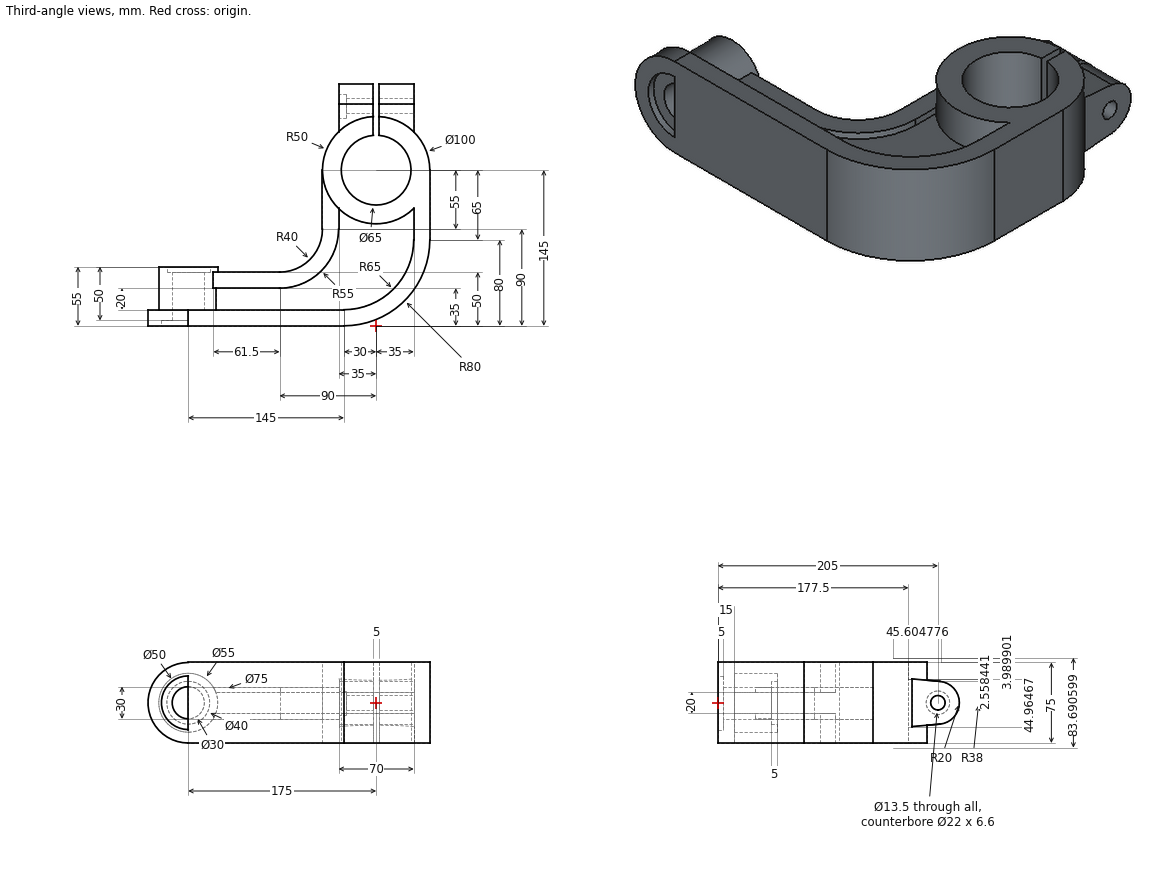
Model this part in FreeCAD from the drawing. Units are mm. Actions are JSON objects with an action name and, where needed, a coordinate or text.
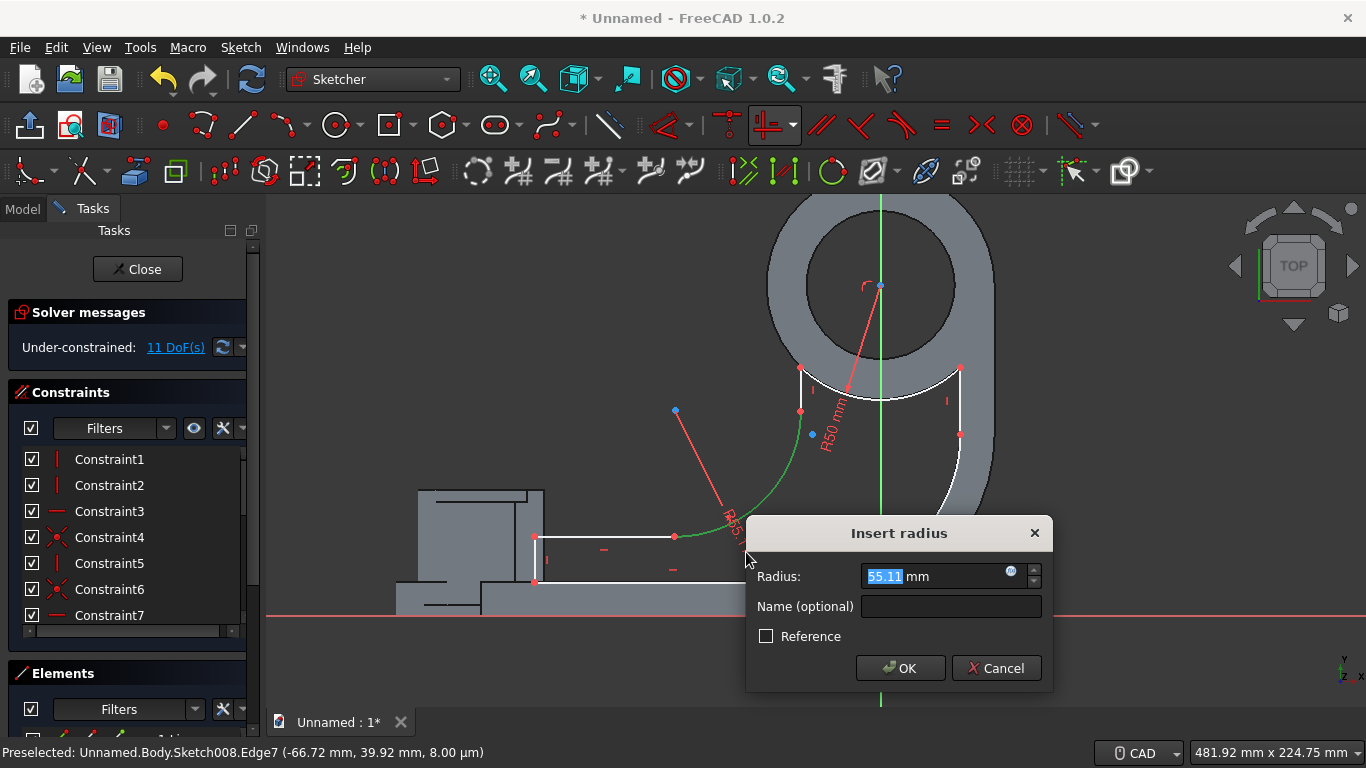
{"action": "type", "text": "55"}
{"action": "key", "text": "Return"}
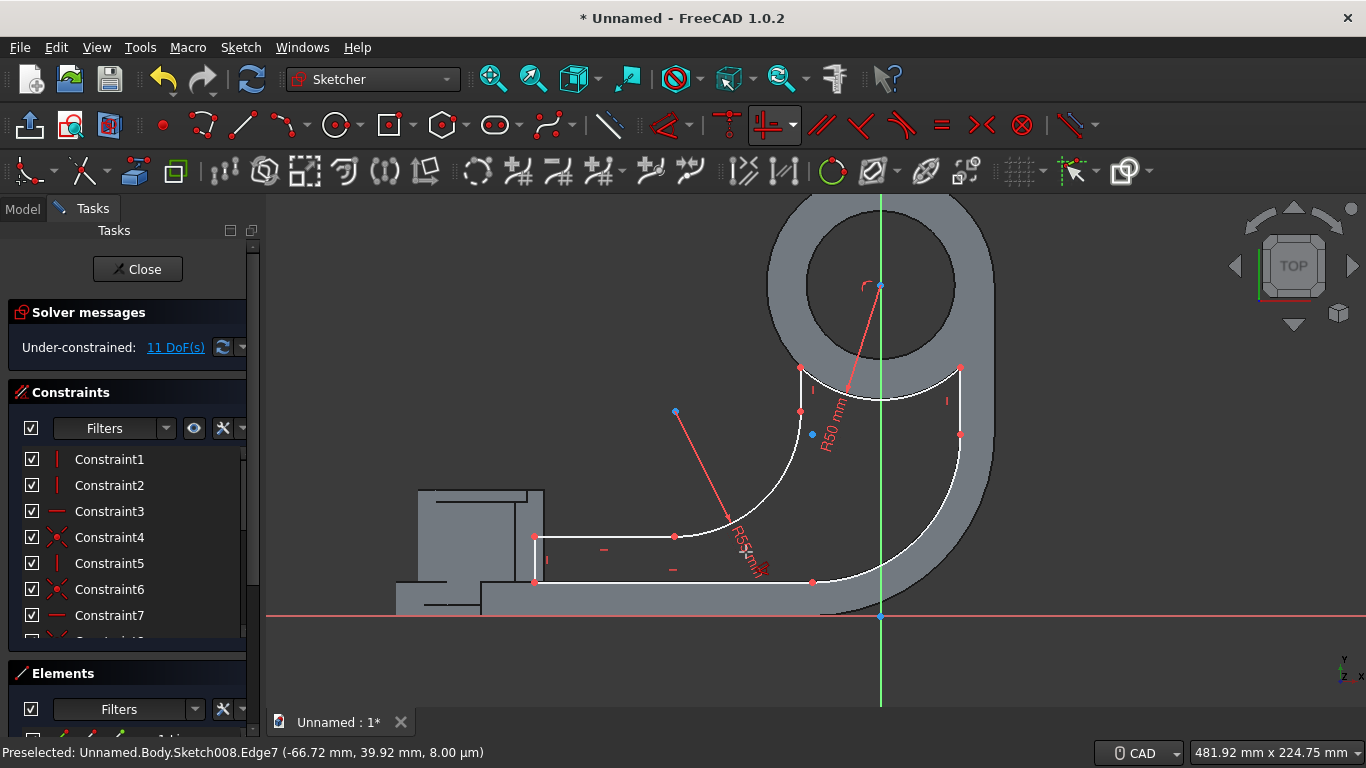
{"action": "left_click", "coordinate": [880, 566]}
{"action": "left_click", "coordinate": [895, 594]}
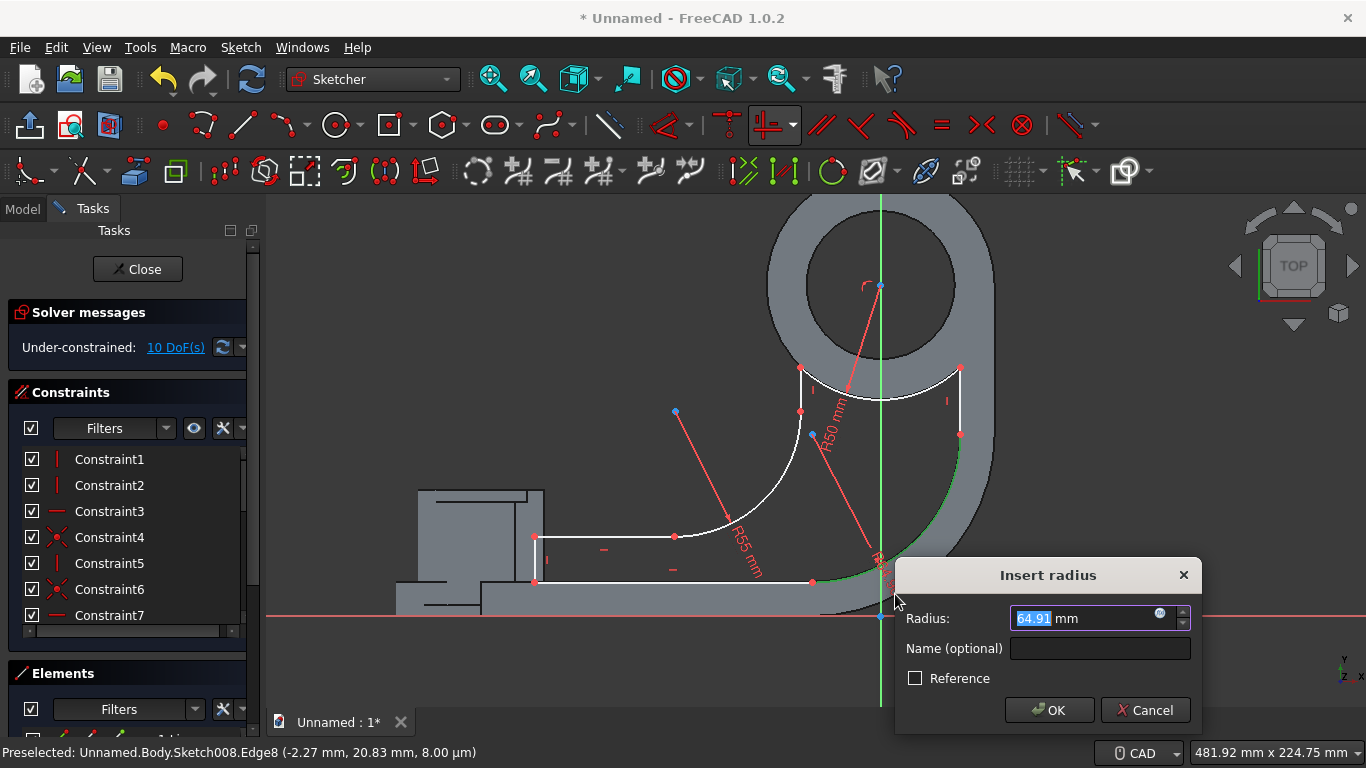
{"action": "type", "text": "65"}
{"action": "key", "text": "Return"}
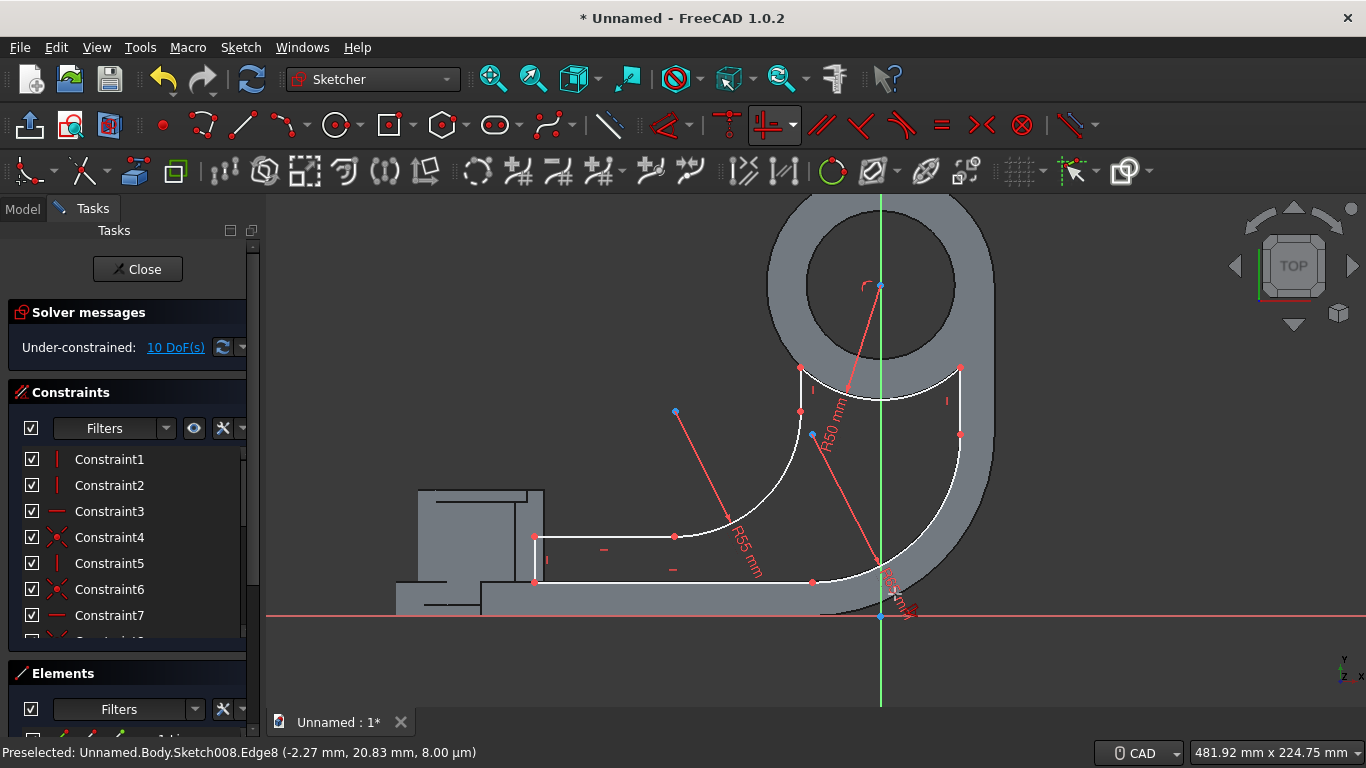
{"action": "left_click", "coordinate": [535, 551]}
{"action": "left_click", "coordinate": [501, 560]}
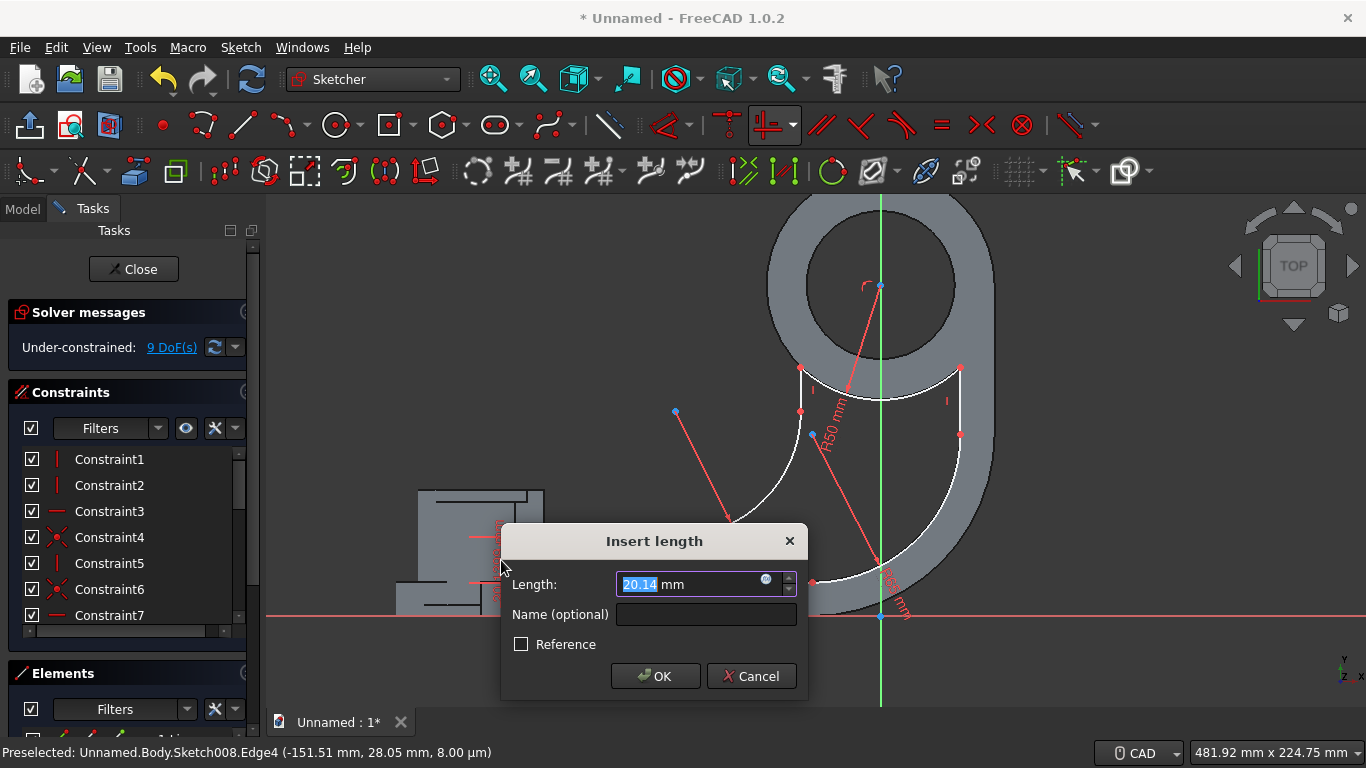
{"action": "type", "text": "20"}
{"action": "key", "text": "Return"}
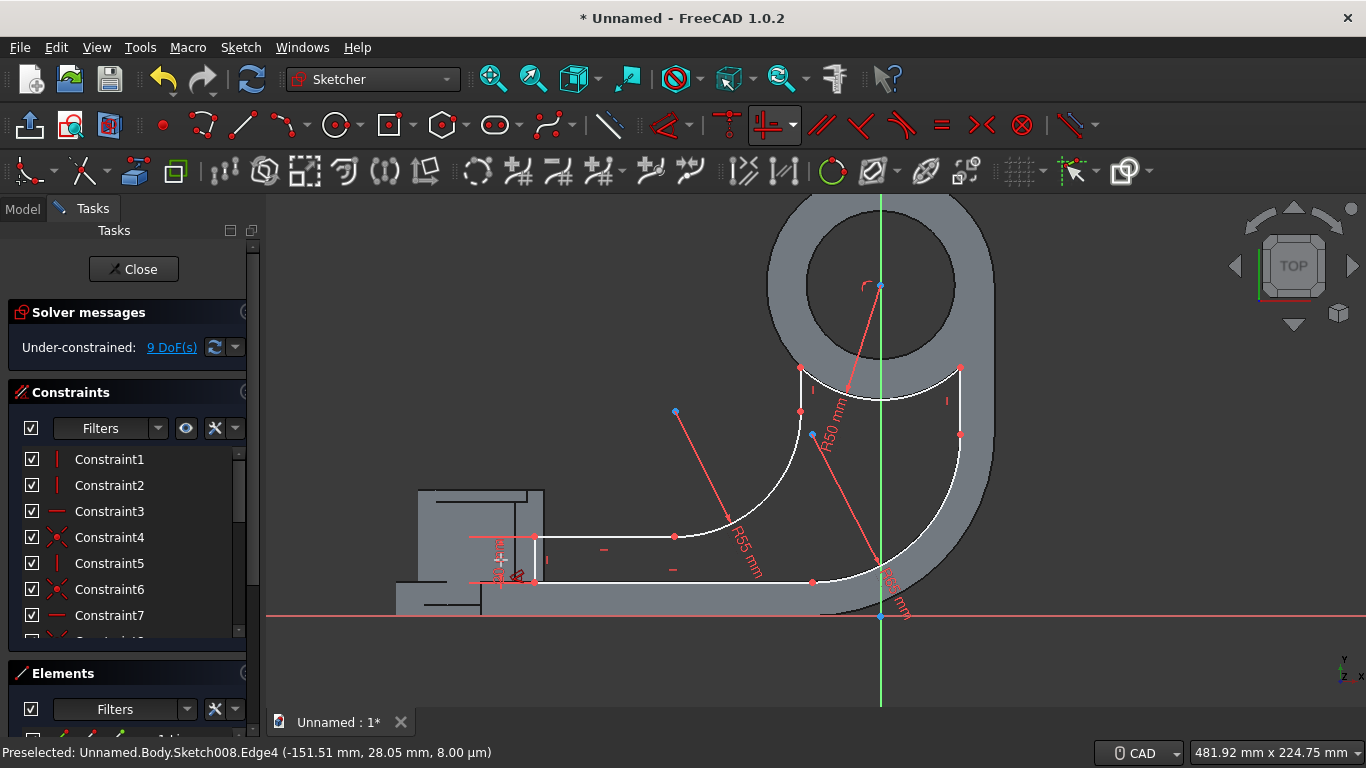
{"action": "left_click", "coordinate": [960, 434]}
{"action": "left_click", "coordinate": [921, 650]}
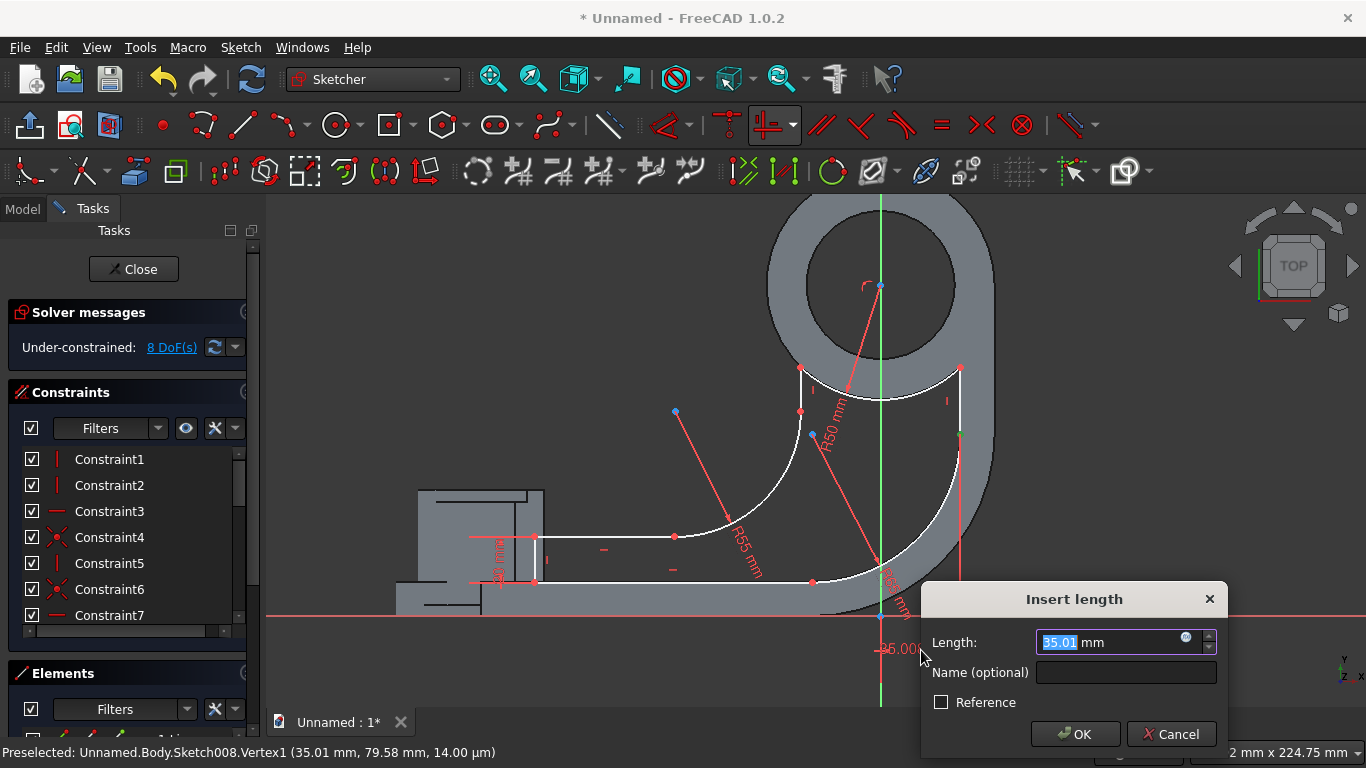
{"action": "type", "text": "35"}
{"action": "key", "text": "Return"}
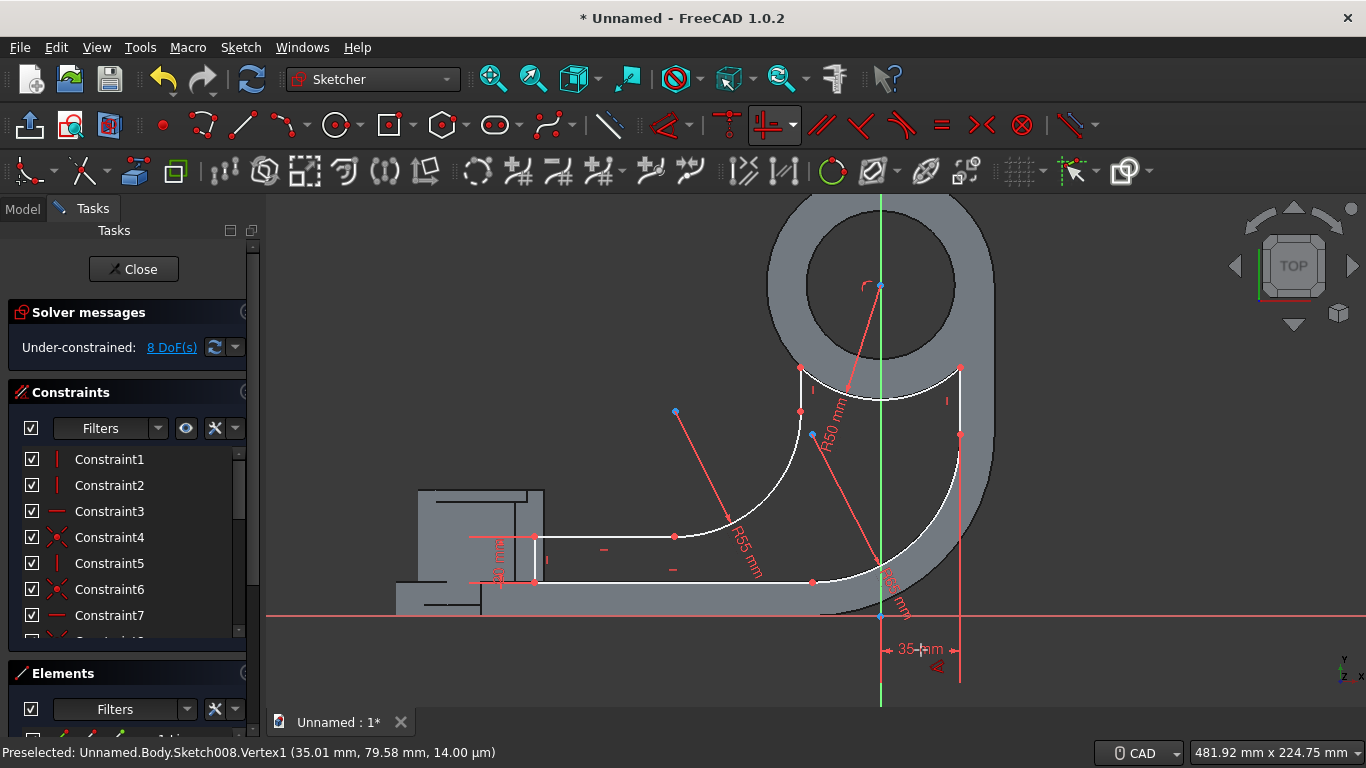
{"action": "left_click", "coordinate": [960, 434]}
{"action": "left_click", "coordinate": [994, 525]}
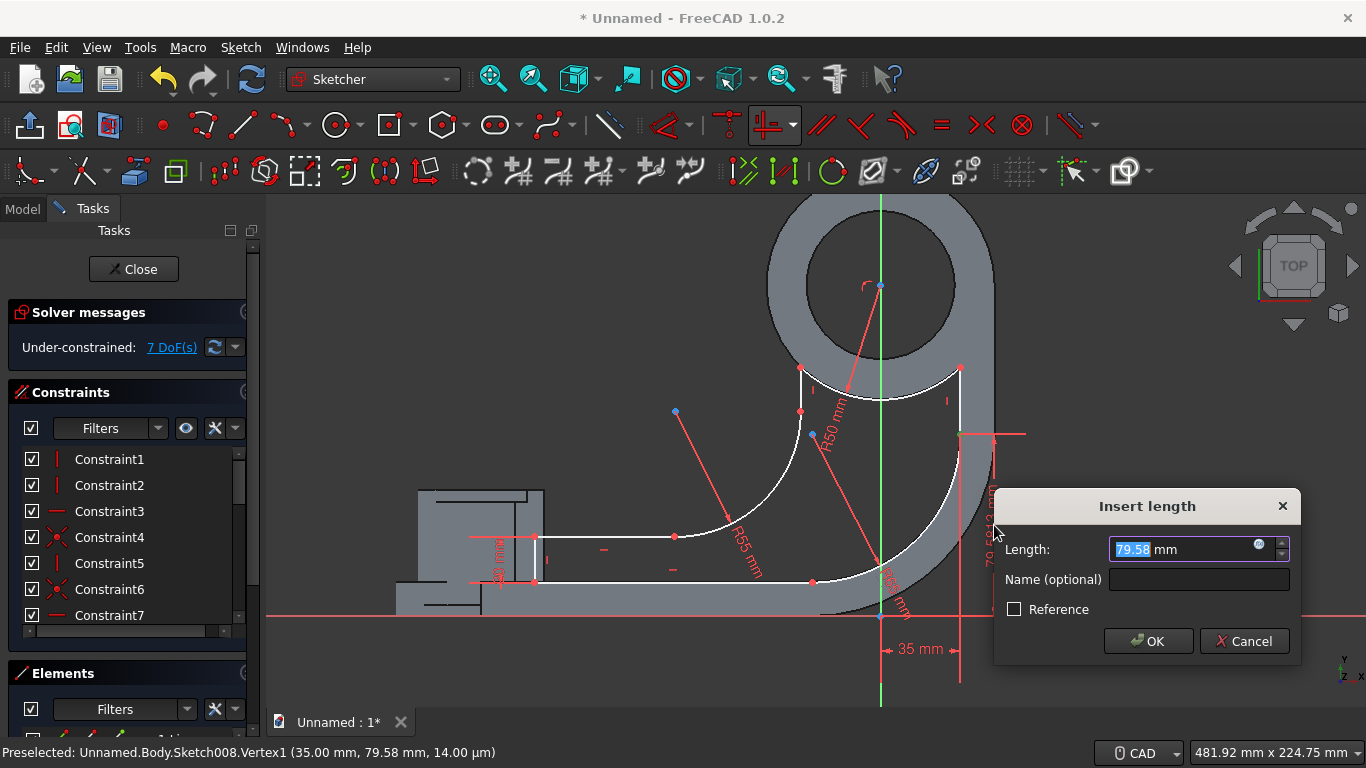
{"action": "type", "text": "80"}
{"action": "key", "text": "Return"}